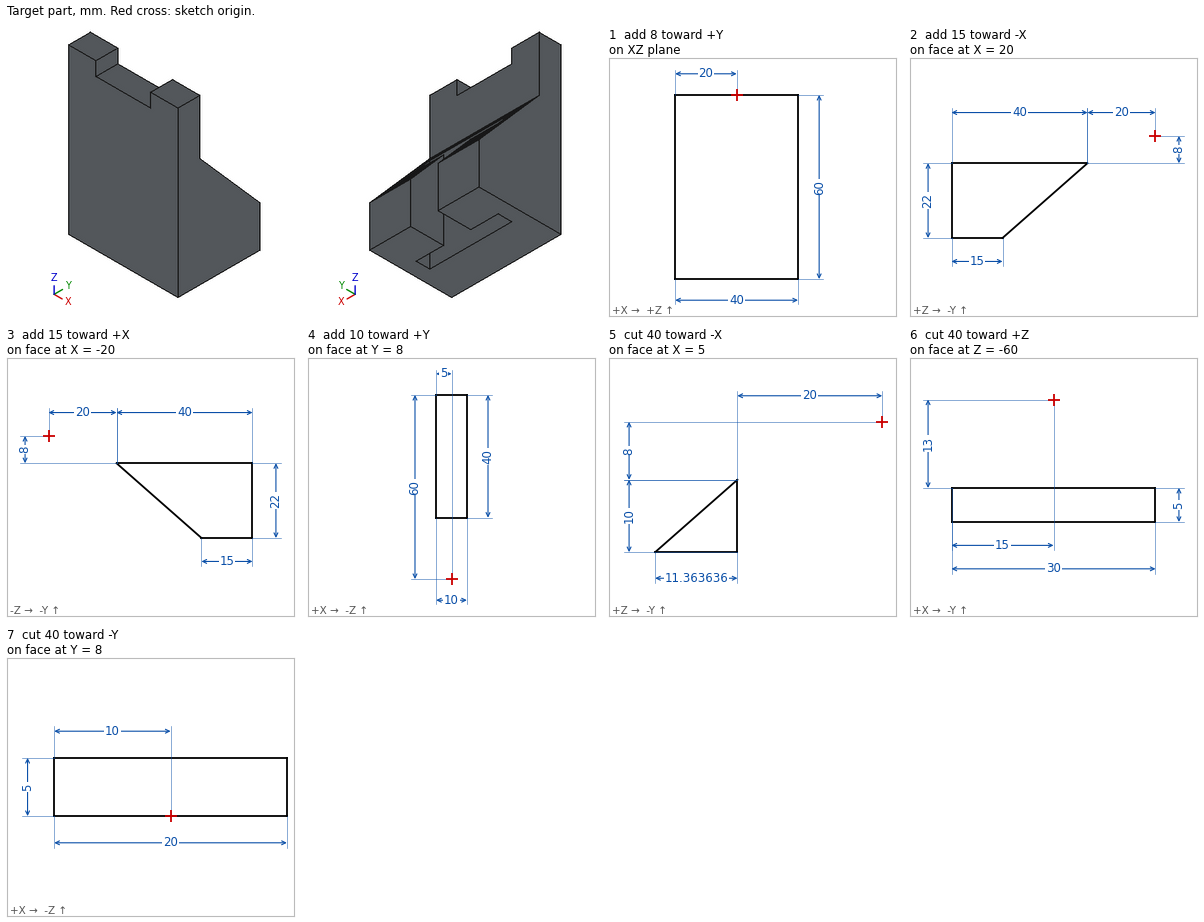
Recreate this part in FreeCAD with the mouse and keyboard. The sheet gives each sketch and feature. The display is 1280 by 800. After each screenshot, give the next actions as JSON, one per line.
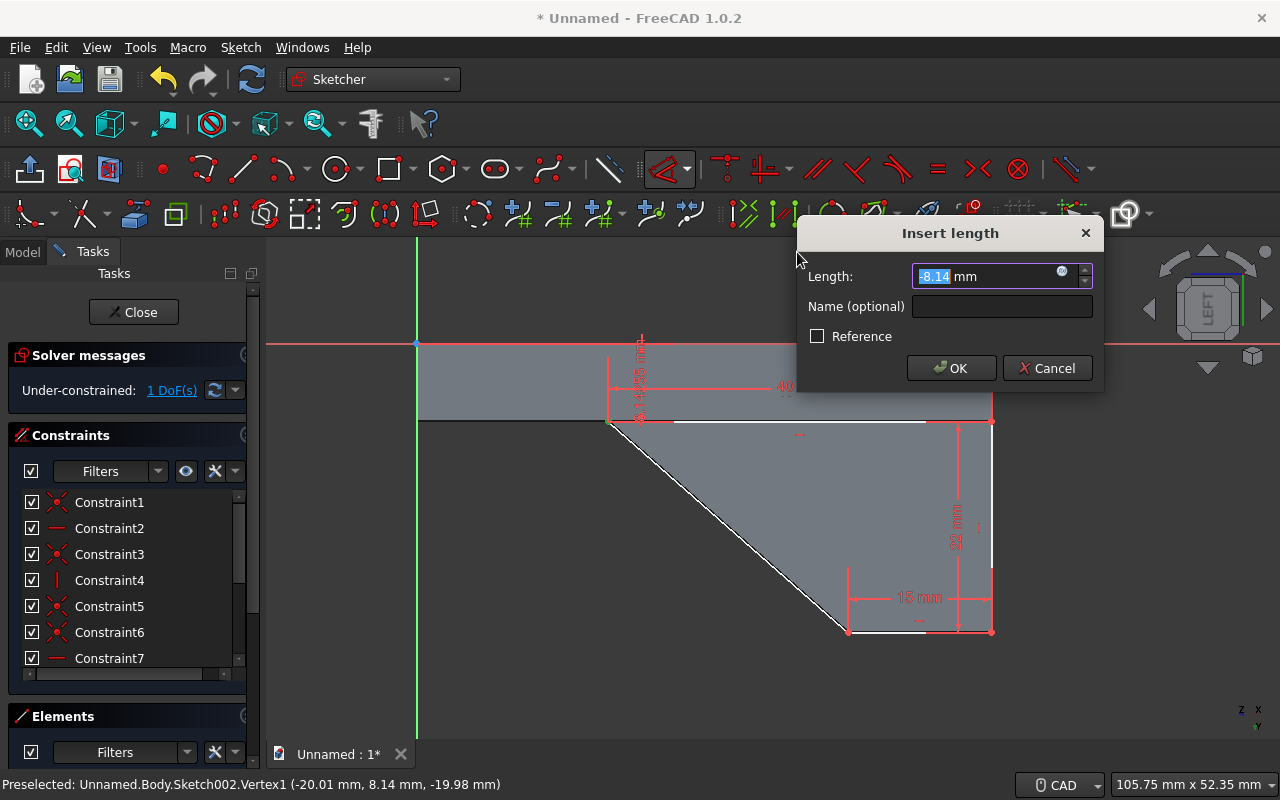
{"action": "type", "text": "-8"}
{"action": "key", "text": "Return"}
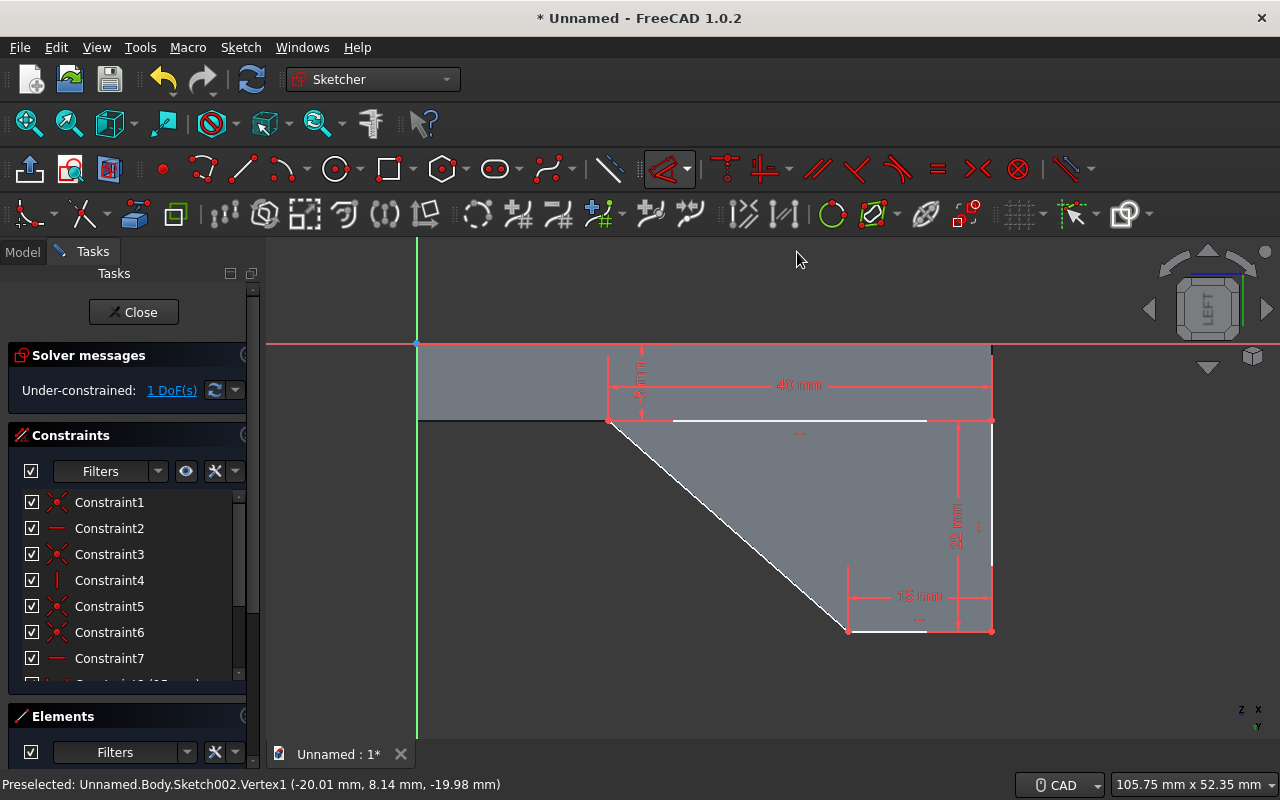
{"action": "left_click", "coordinate": [608, 421]}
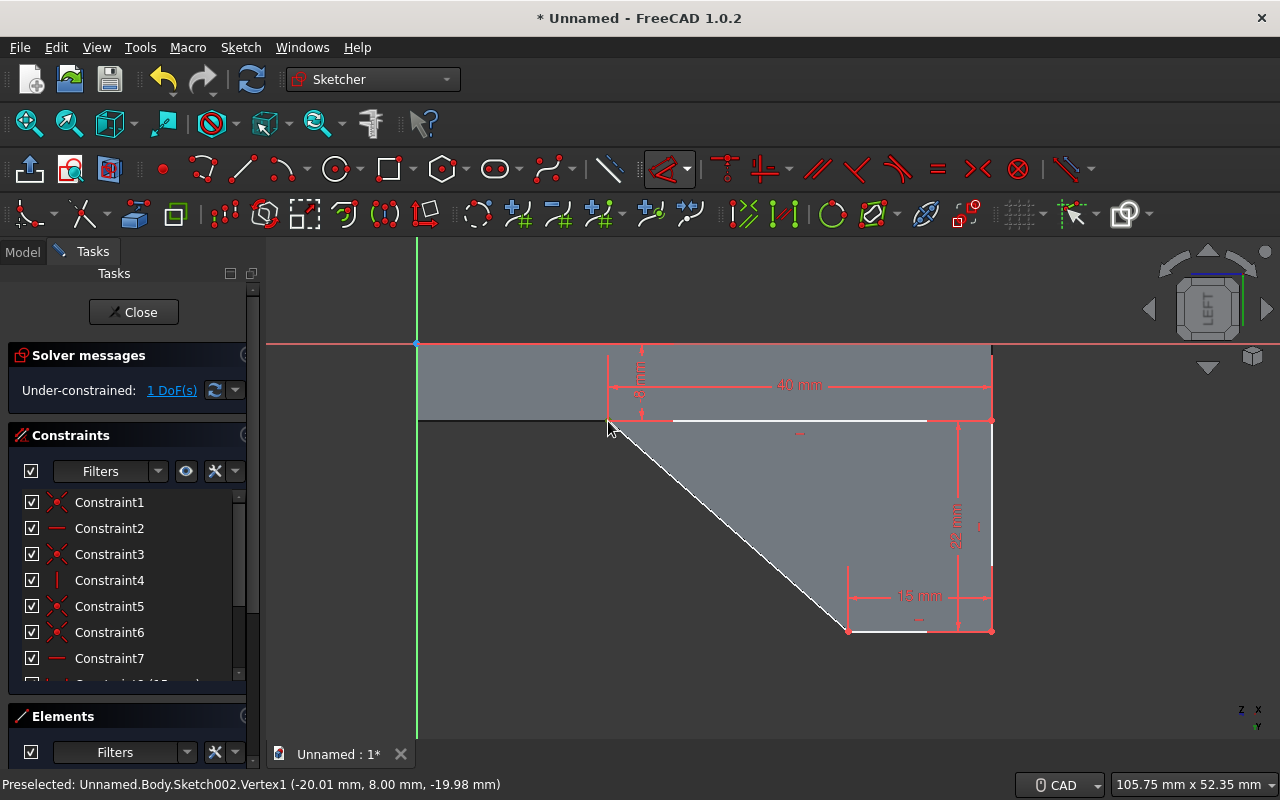
{"action": "left_click", "coordinate": [690, 170]}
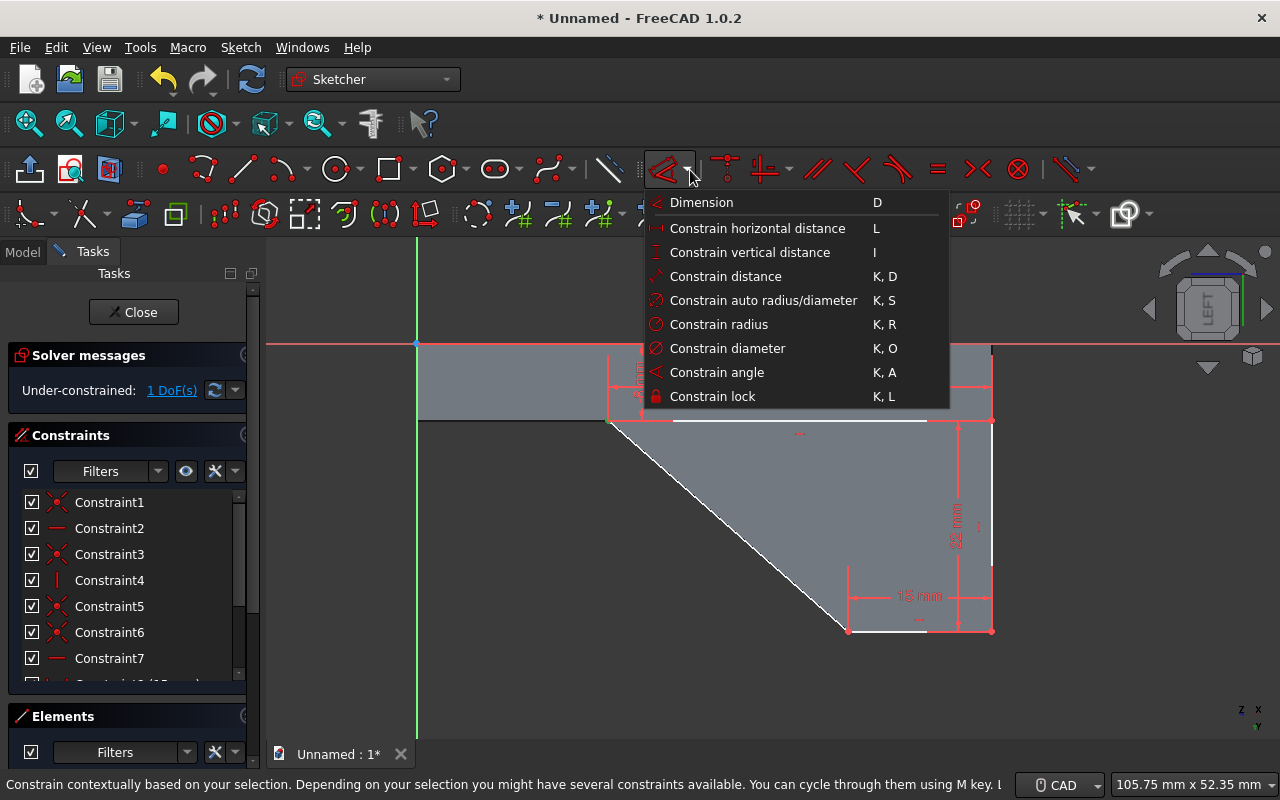
{"action": "left_click", "coordinate": [797, 228]}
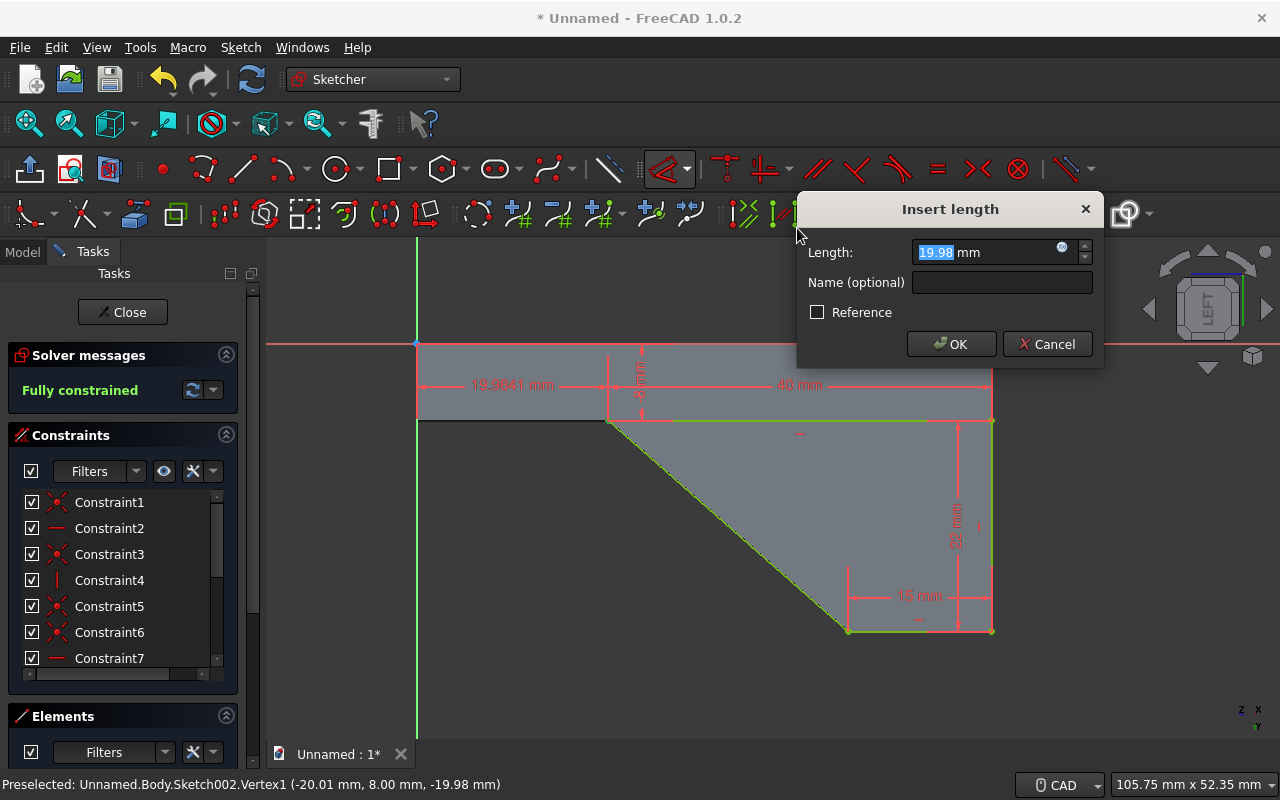
{"action": "type", "text": "20"}
{"action": "key", "text": "Return"}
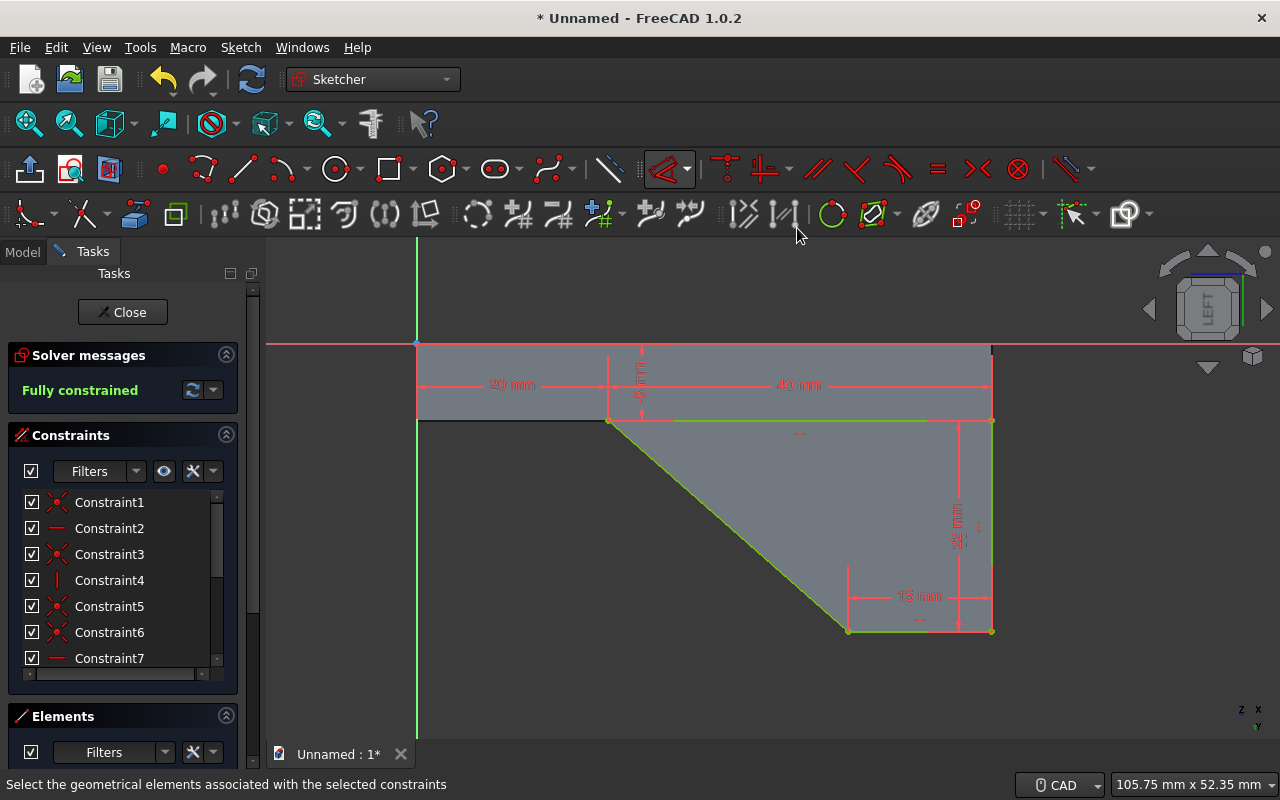
{"action": "left_click", "coordinate": [123, 312]}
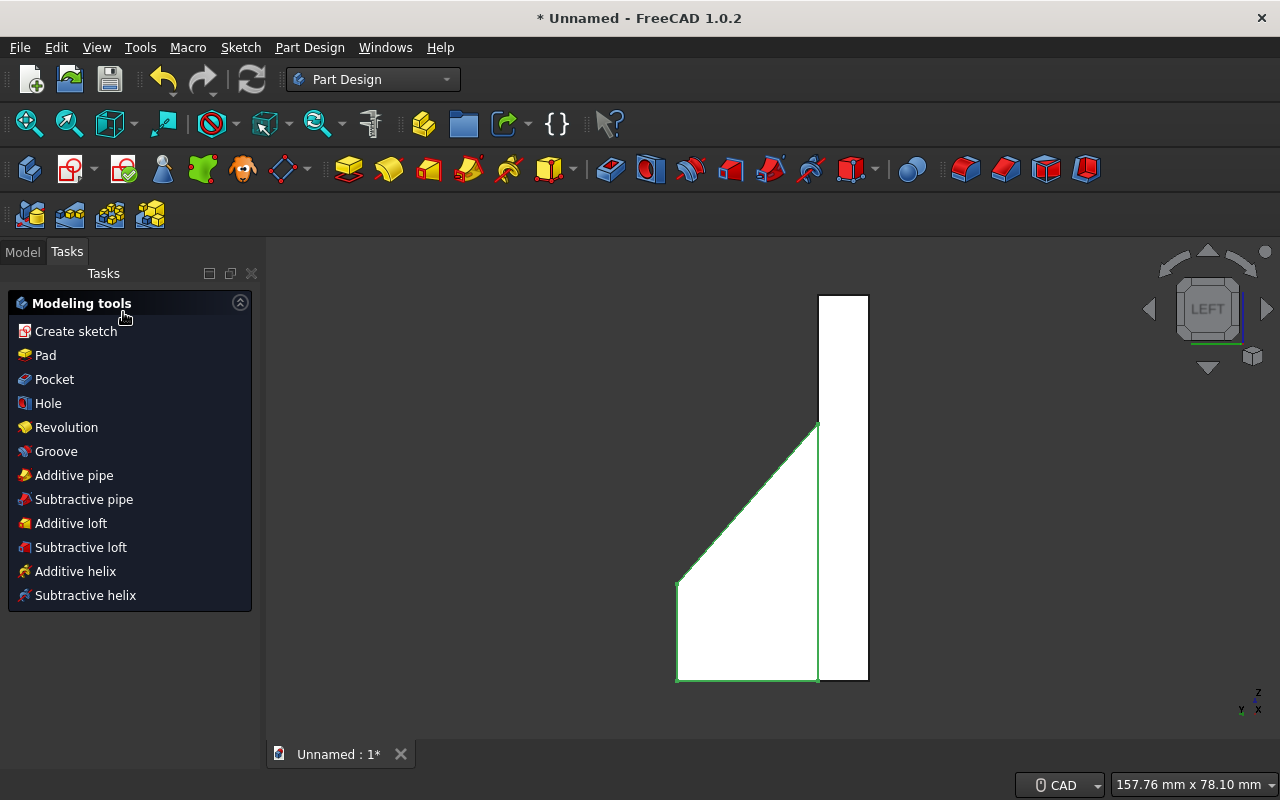
{"action": "left_click", "coordinate": [350, 170]}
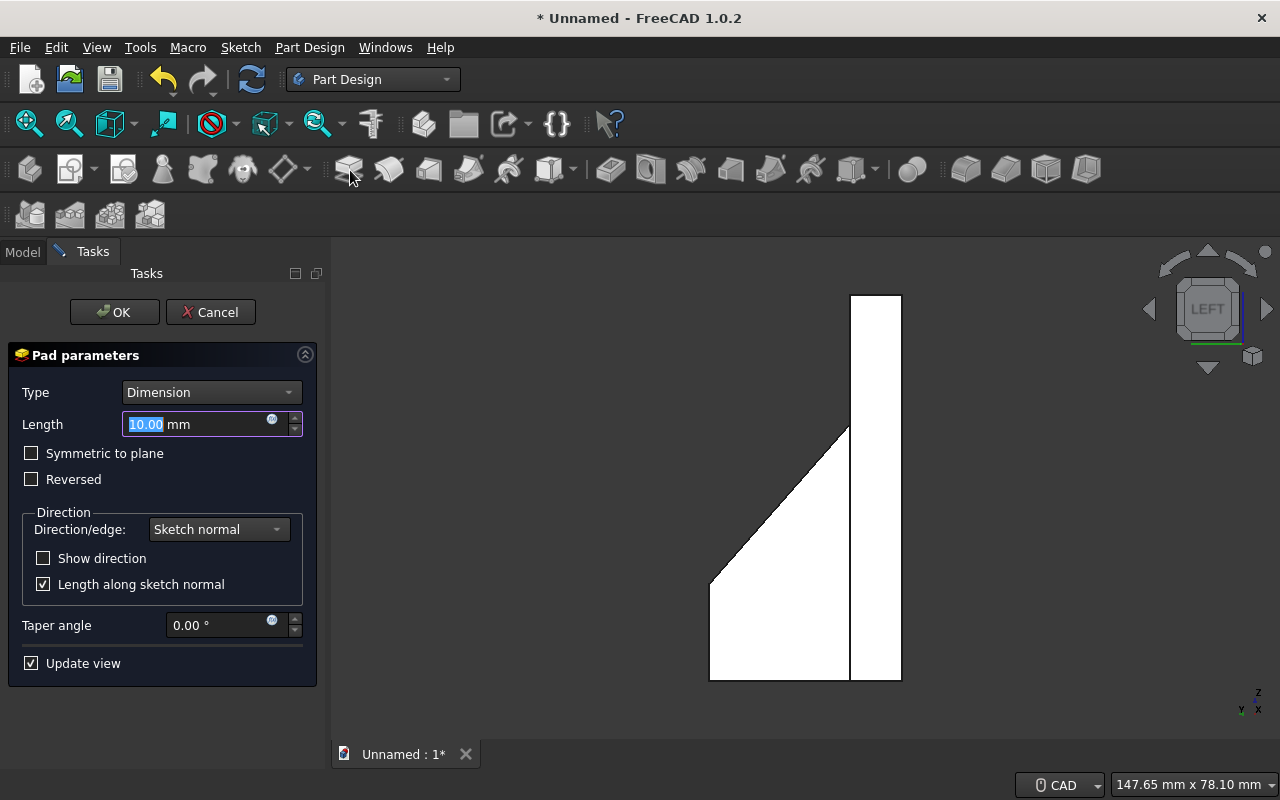
{"action": "type", "text": "15"}
{"action": "key", "text": "Tab"}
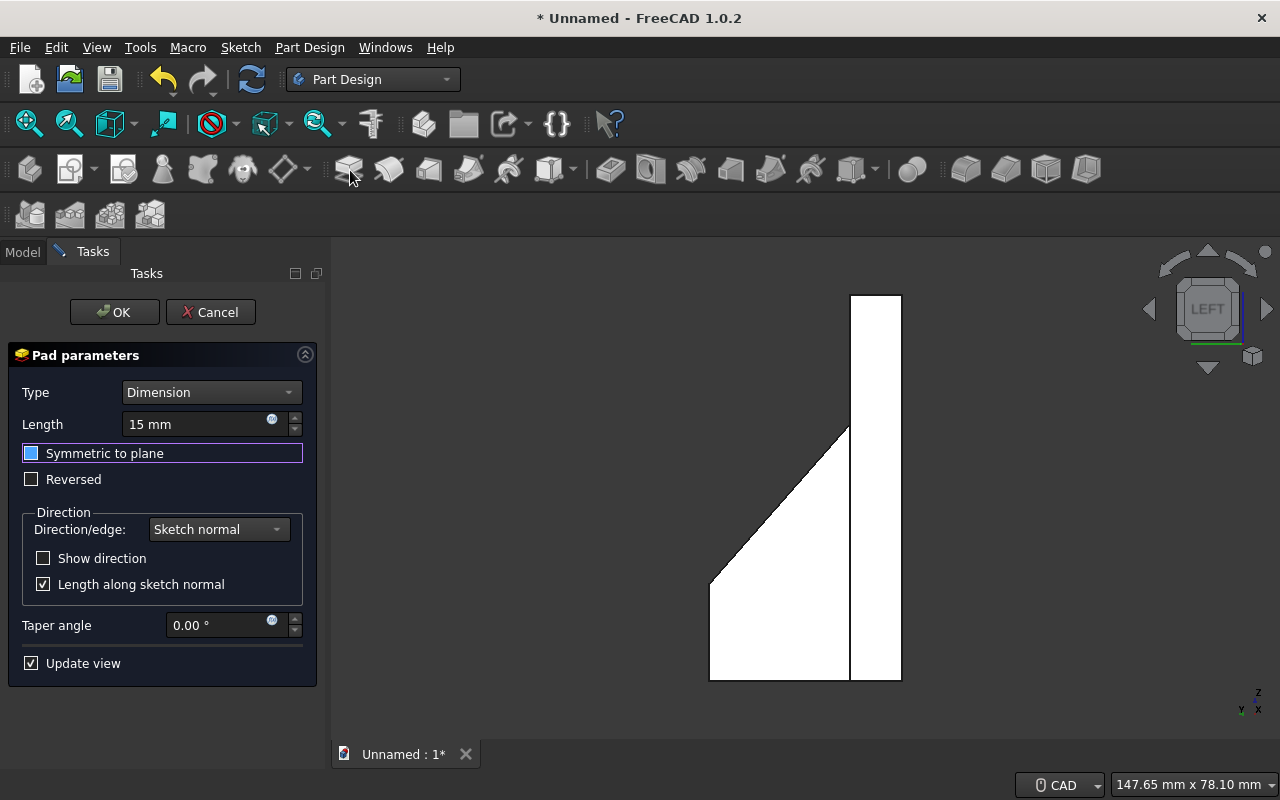
{"action": "left_click", "coordinate": [30, 479]}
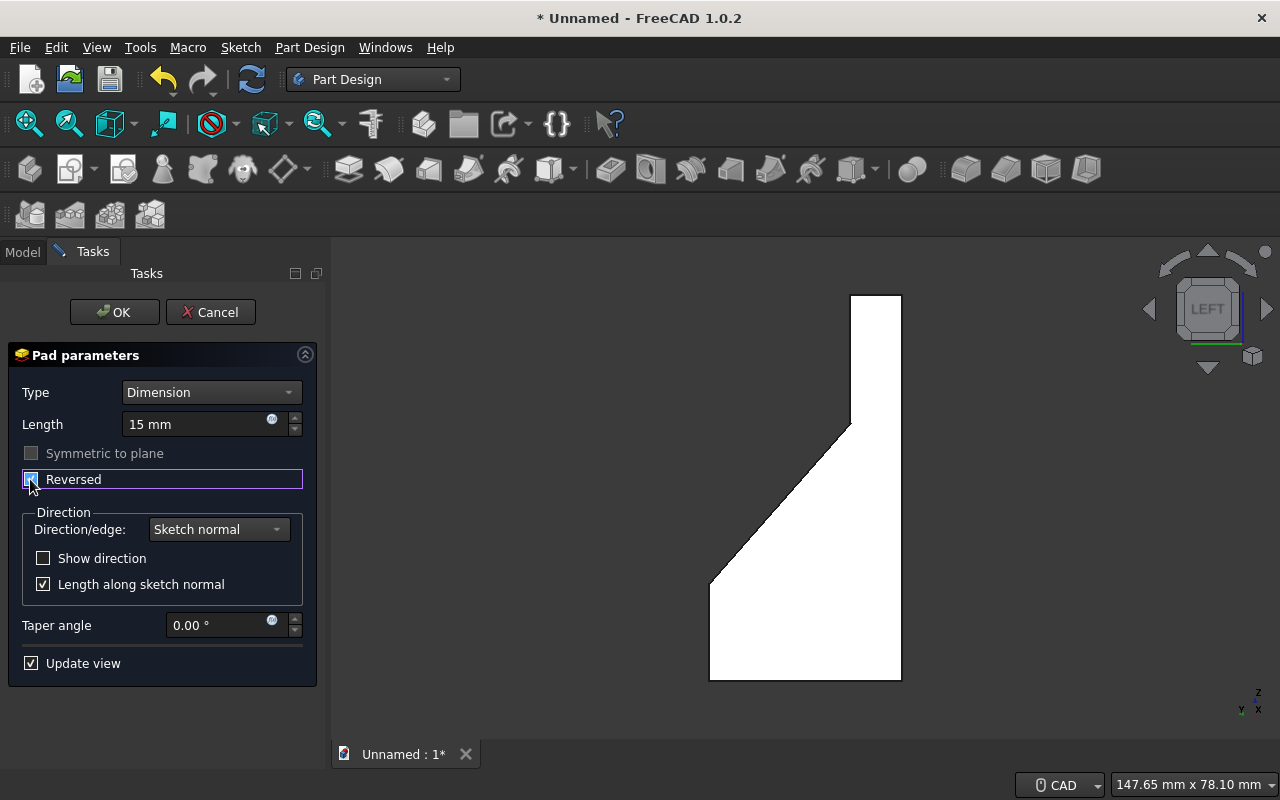
{"action": "left_click", "coordinate": [115, 312]}